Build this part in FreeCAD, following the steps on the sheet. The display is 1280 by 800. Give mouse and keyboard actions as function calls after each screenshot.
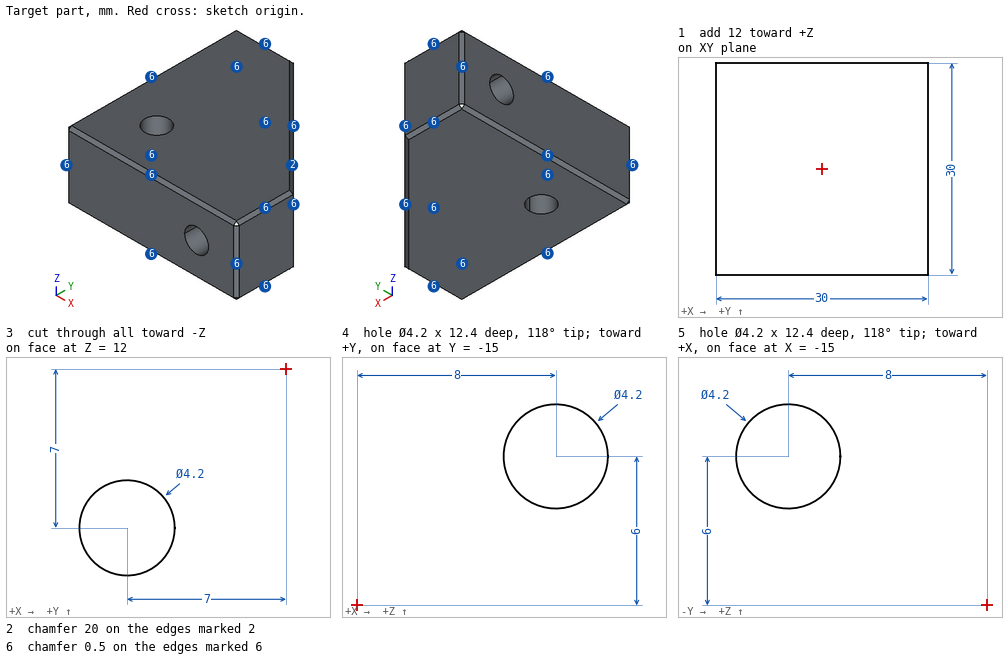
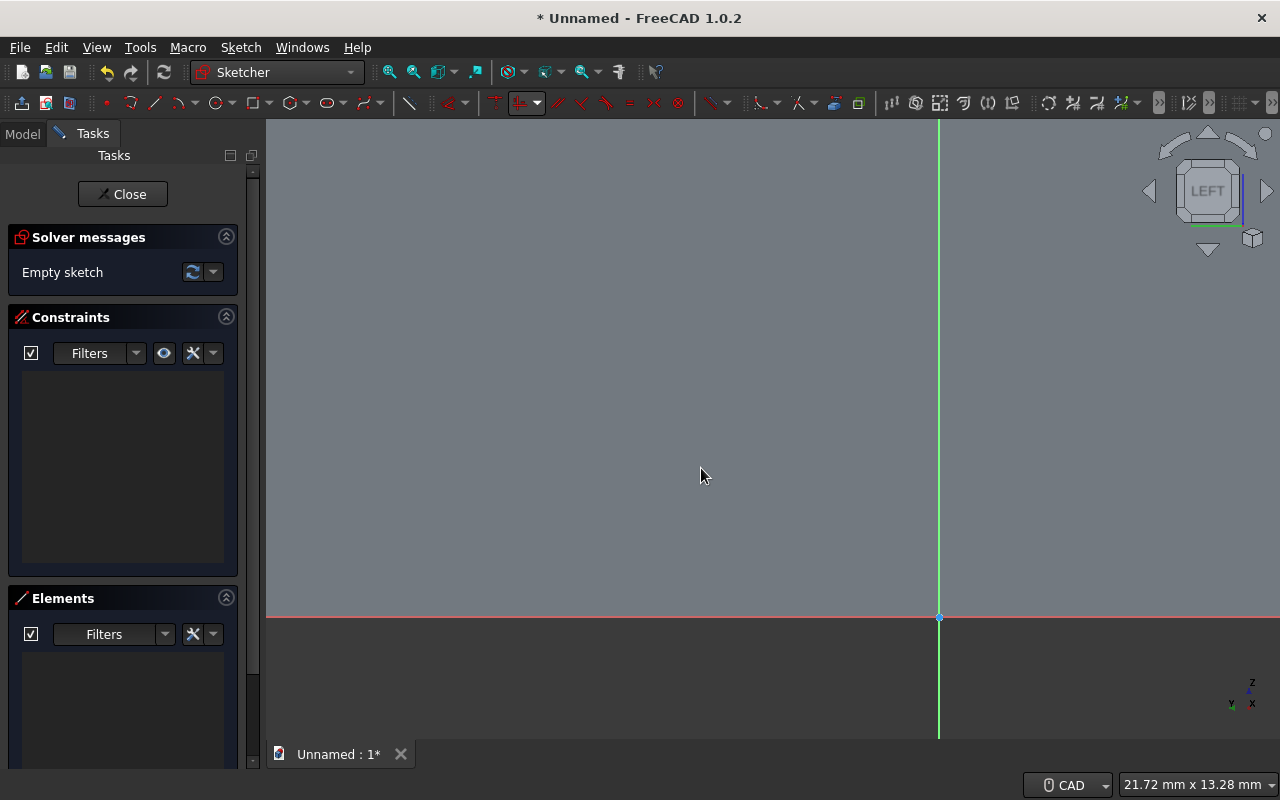
click(216, 104)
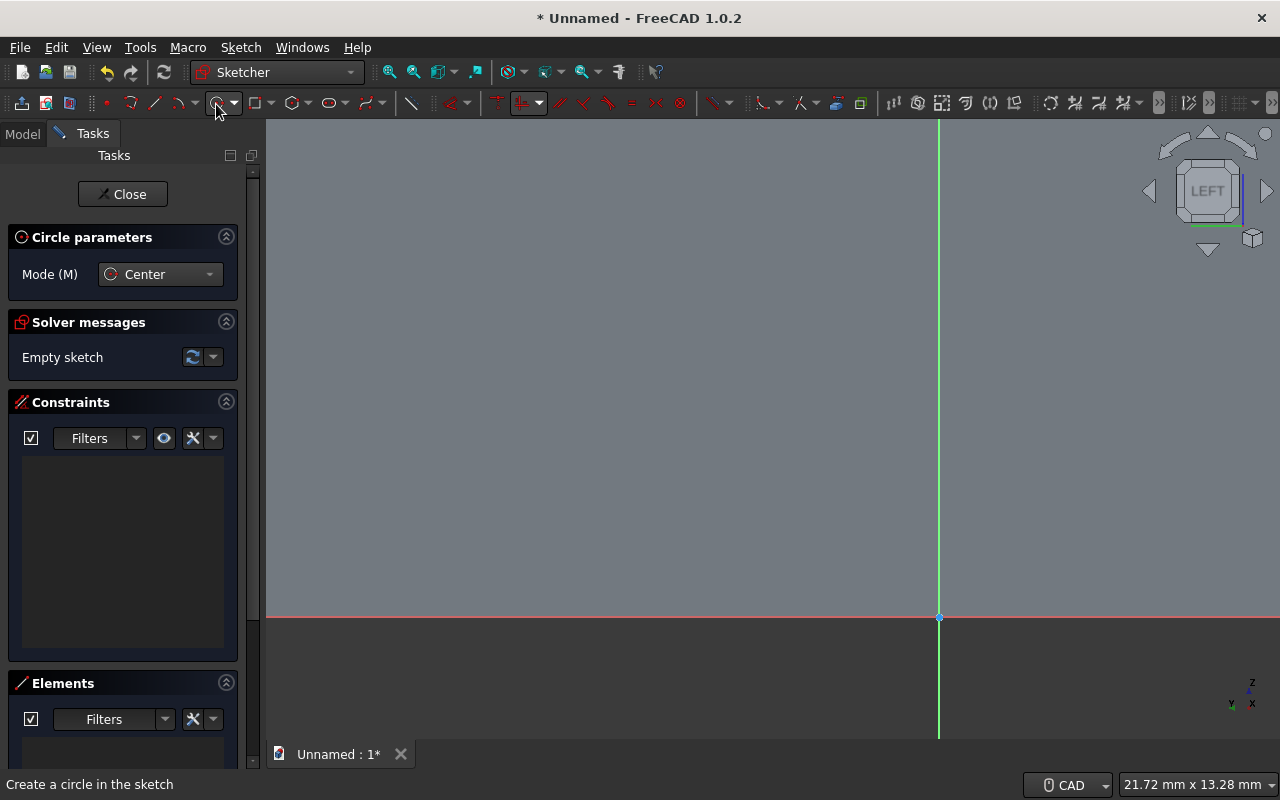
click(566, 337)
click(635, 268)
key(Escape)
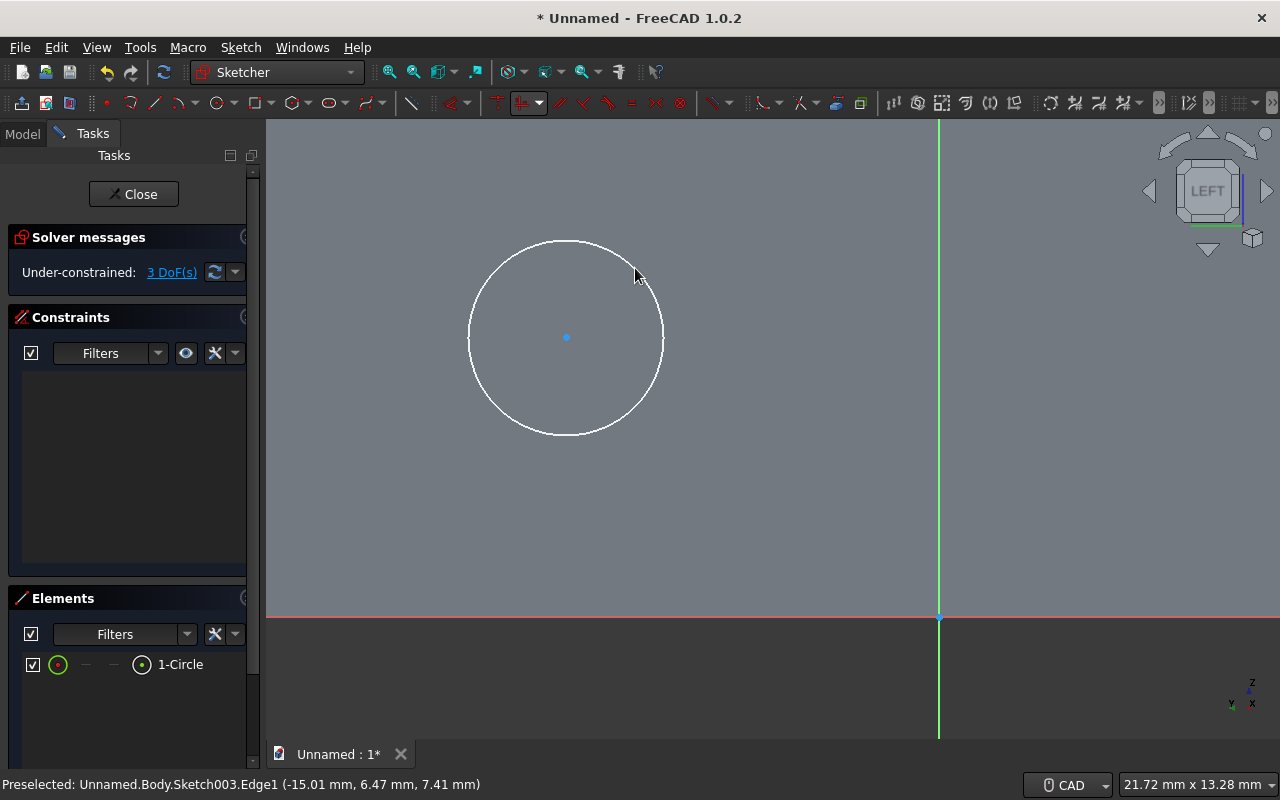
click(450, 104)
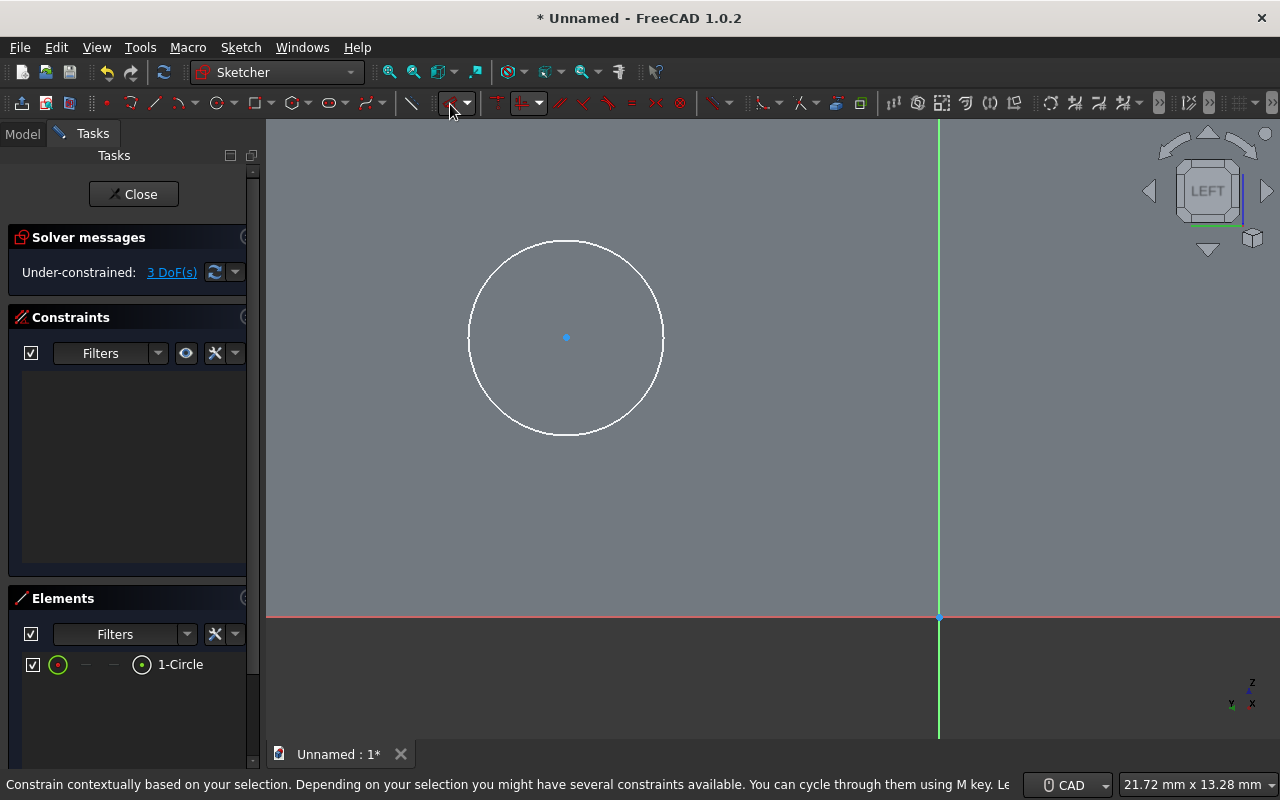
click(635, 269)
click(658, 246)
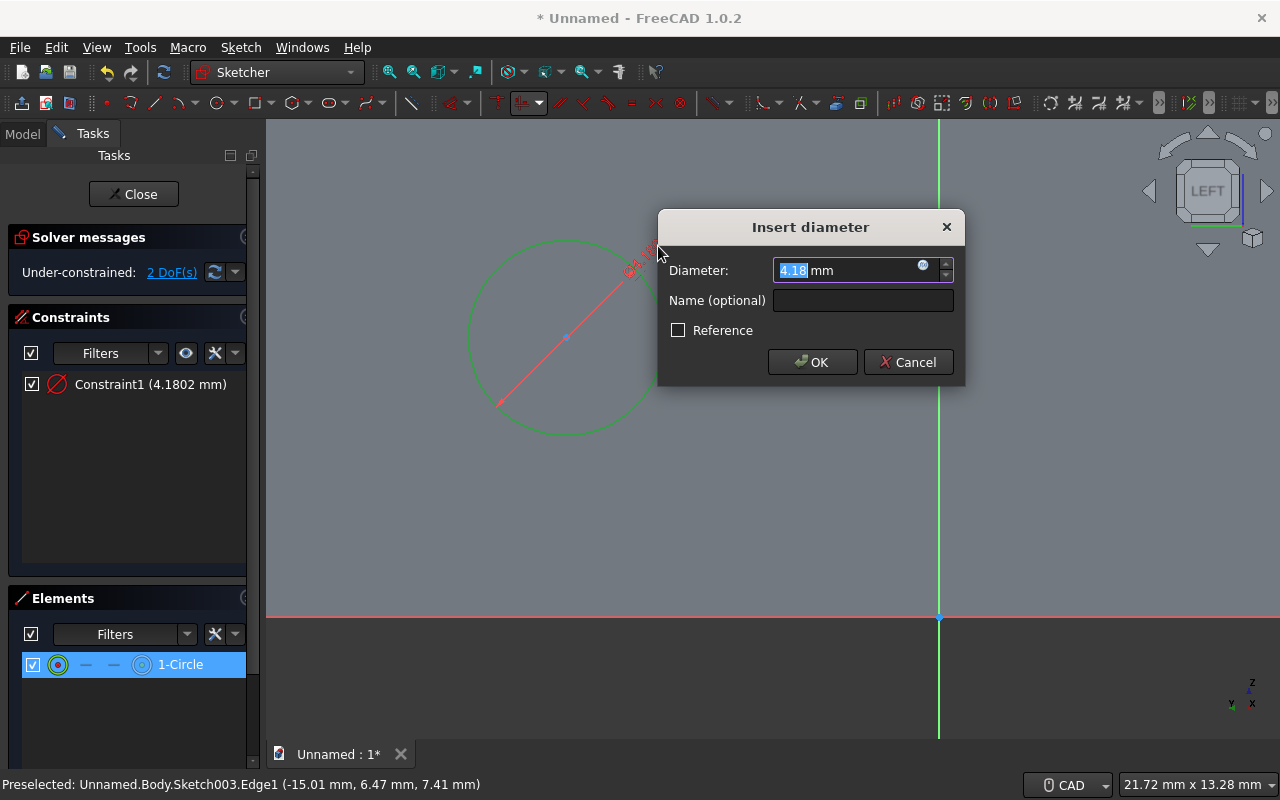
text(4.2)
key(Return)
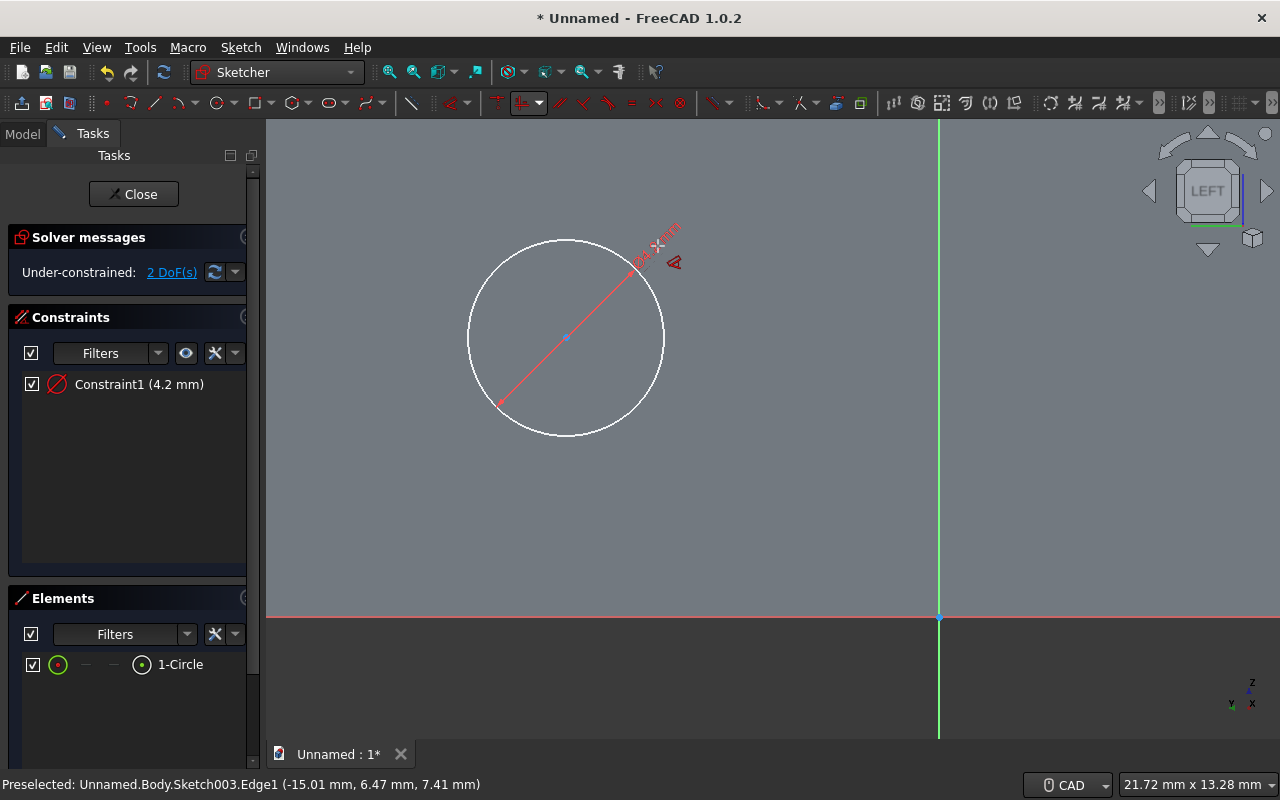
click(566, 338)
click(753, 651)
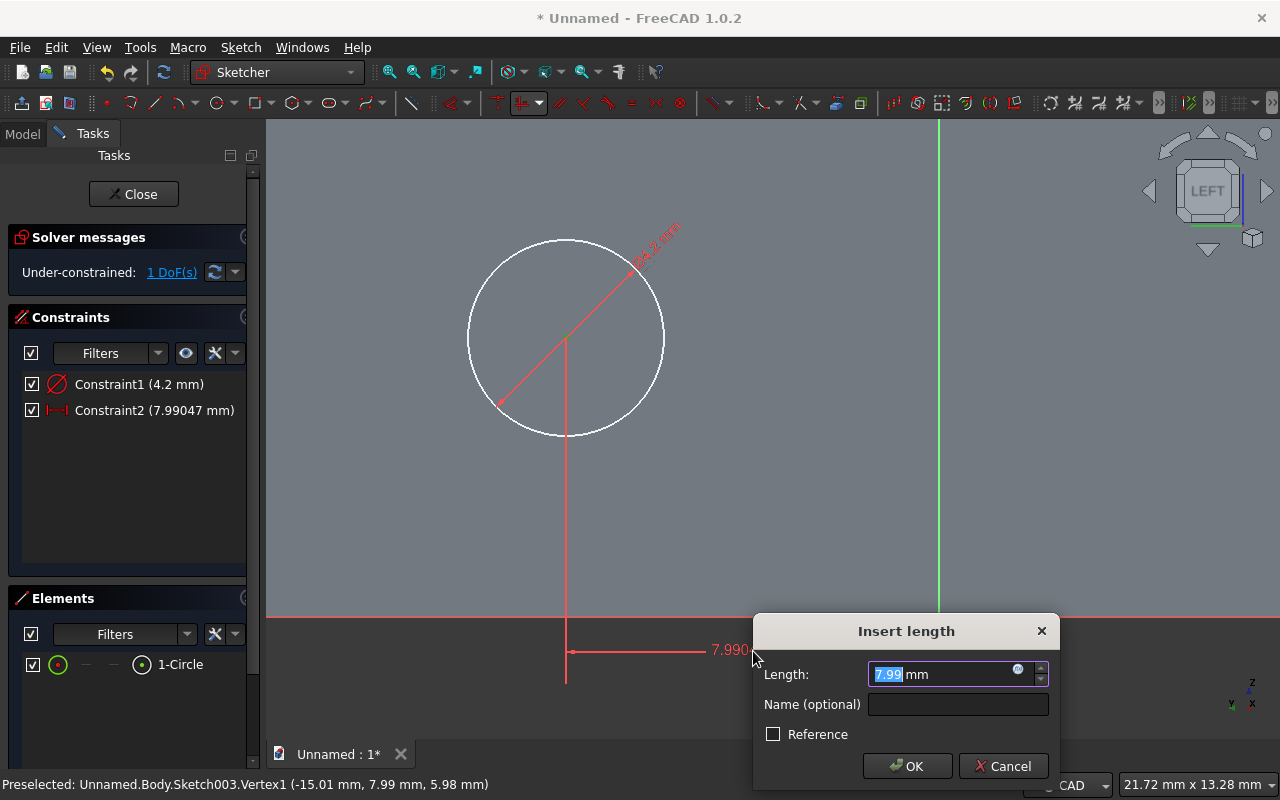
text(8)
key(Return)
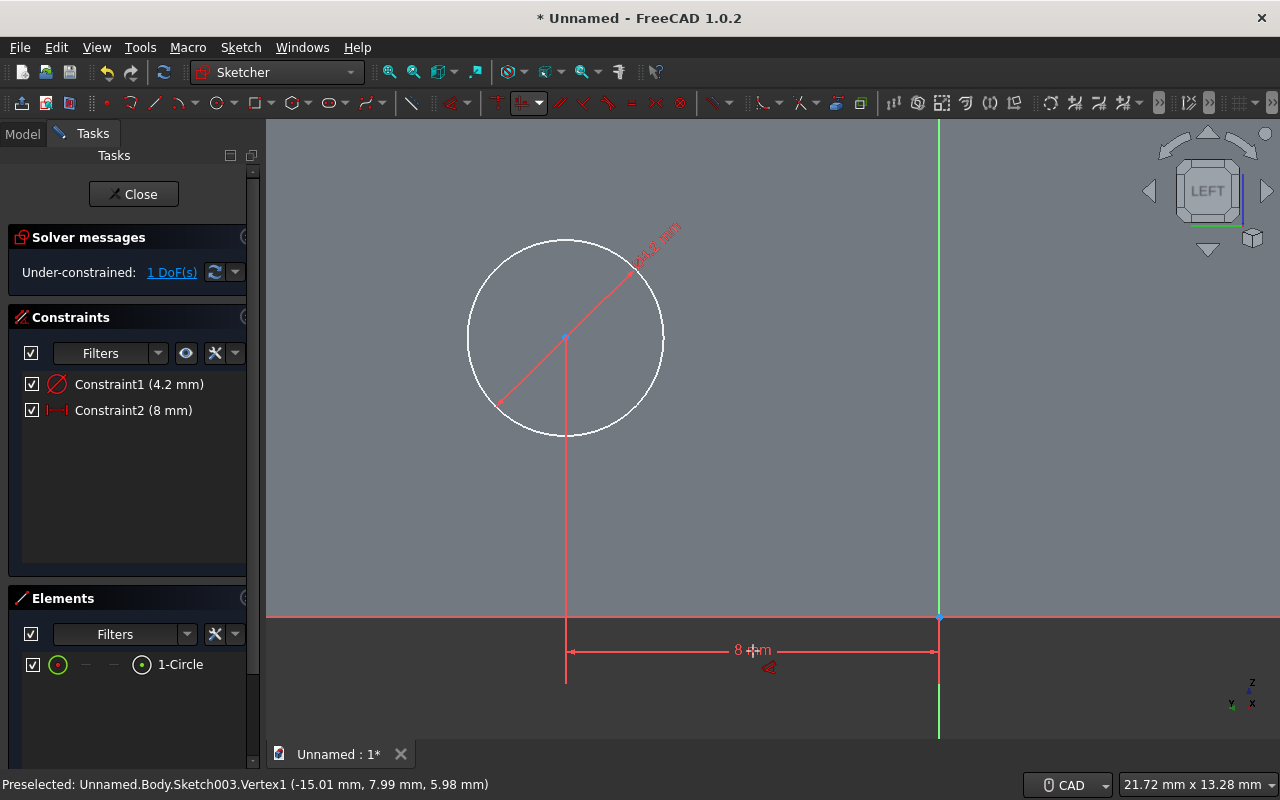
click(566, 338)
click(973, 478)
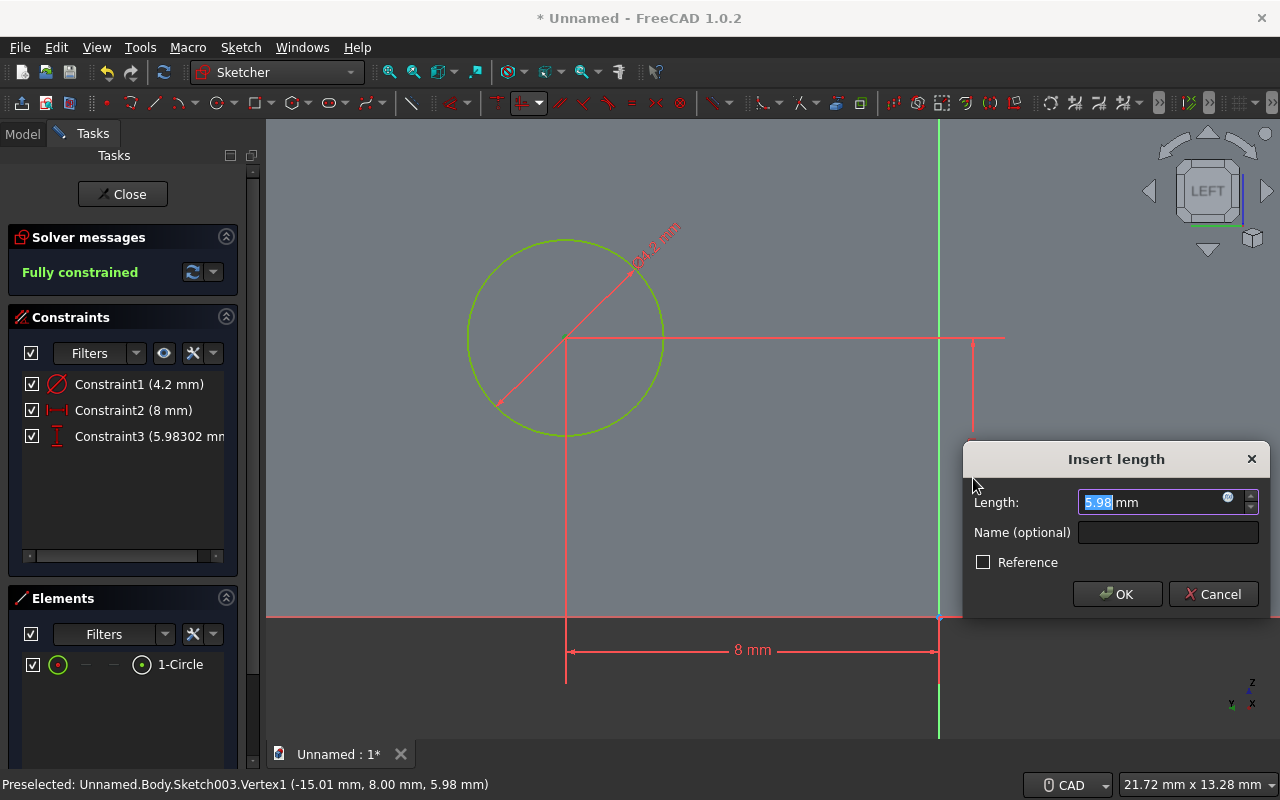
text(6)
key(Return)
key(Escape)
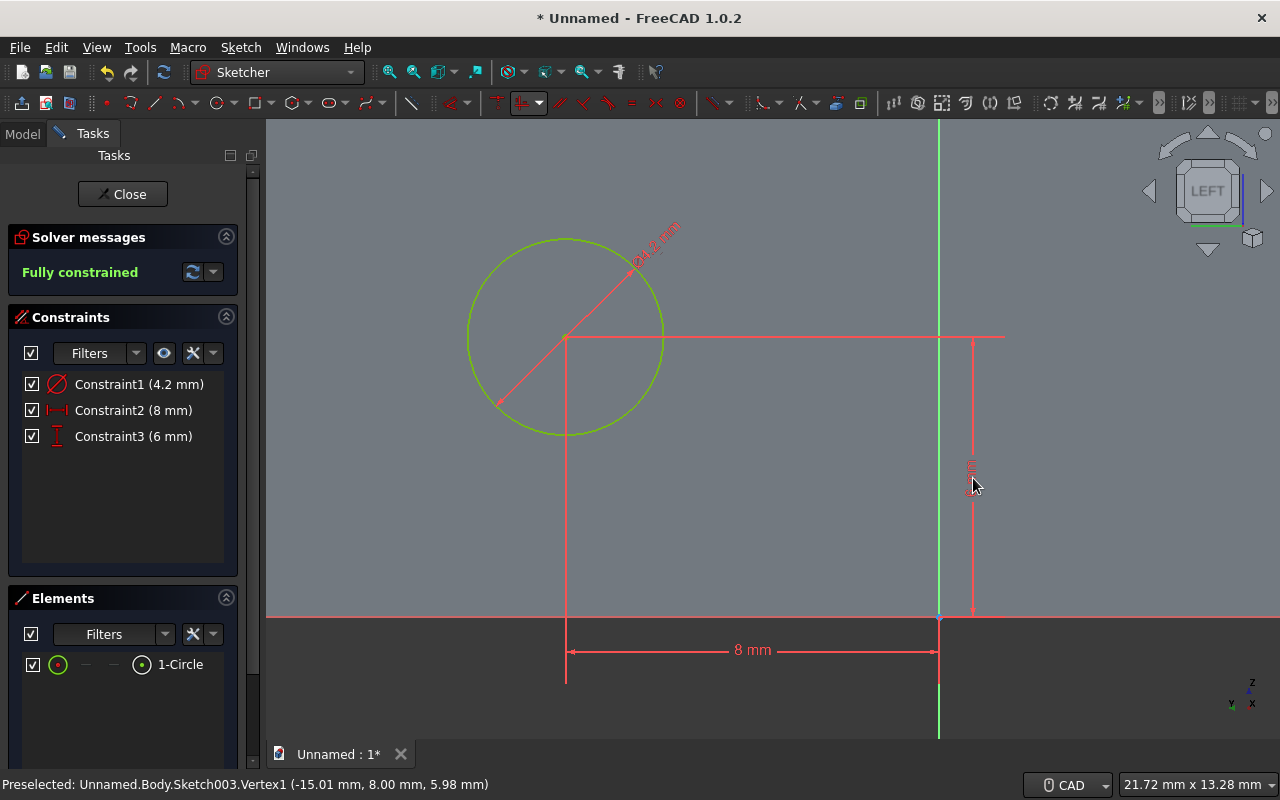
click(123, 194)